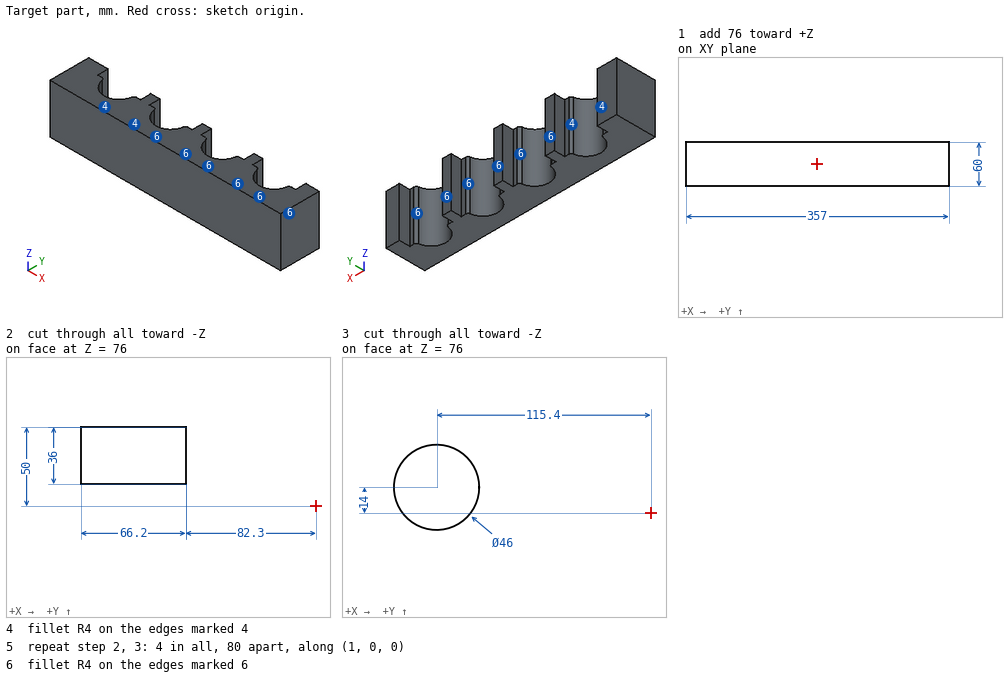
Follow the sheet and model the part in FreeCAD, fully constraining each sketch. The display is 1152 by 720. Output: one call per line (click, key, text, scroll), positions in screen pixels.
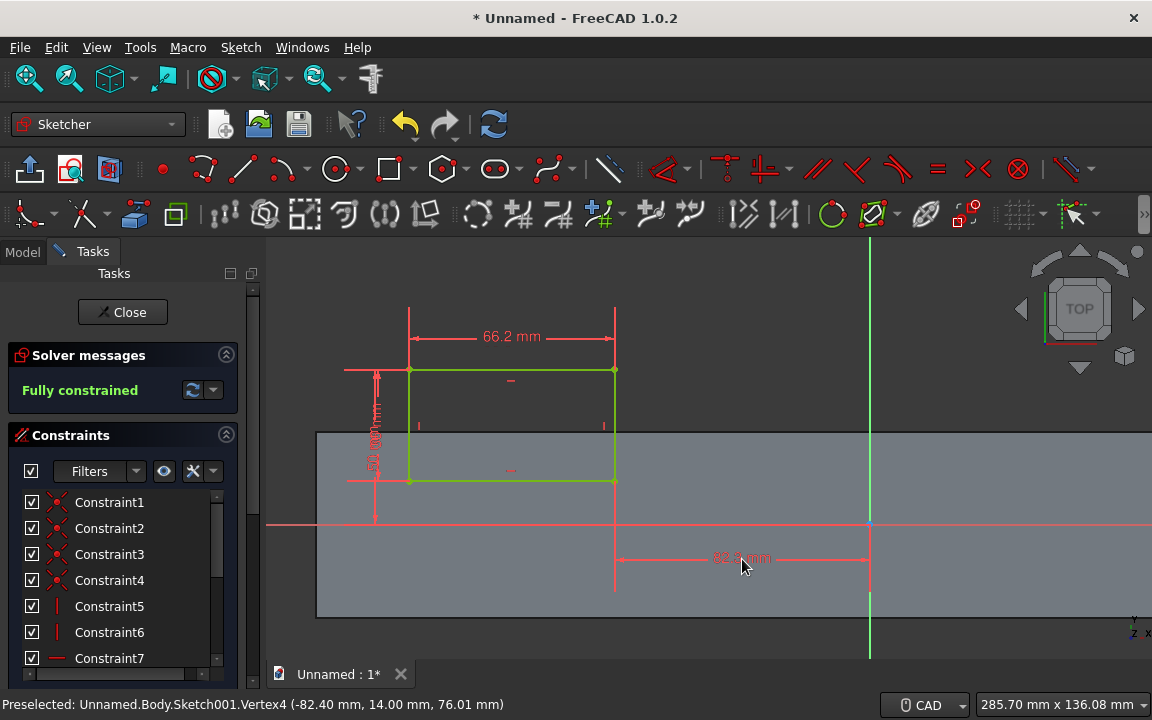
click(123, 312)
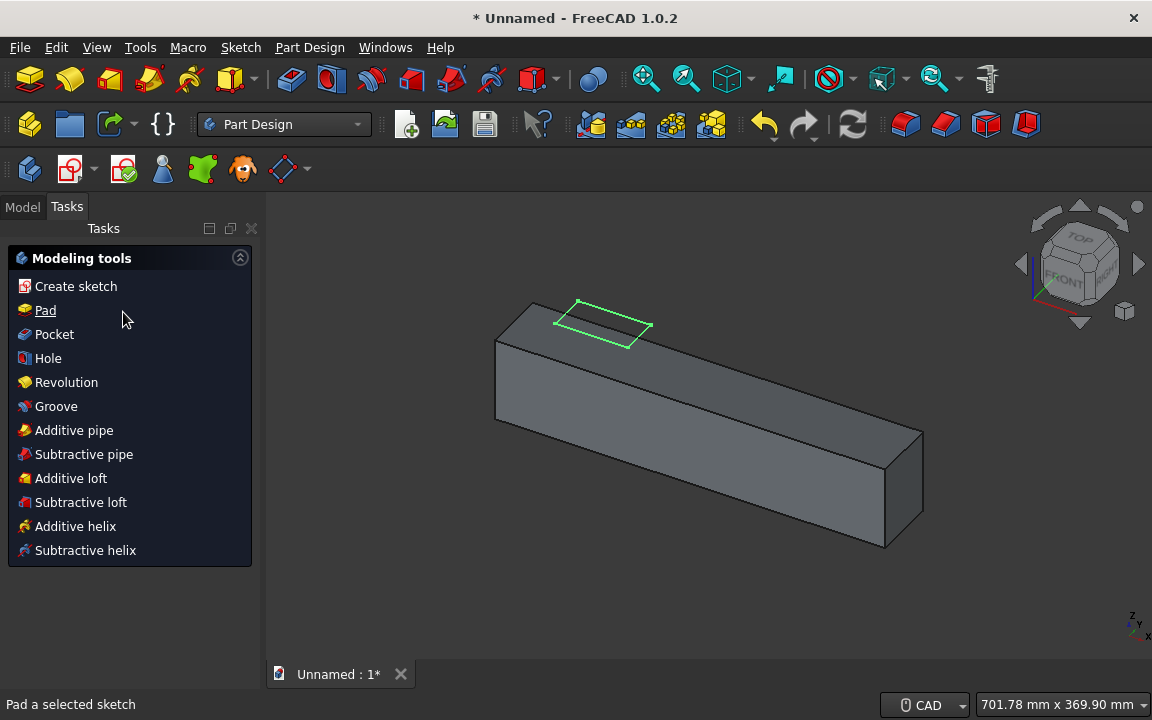
click(292, 80)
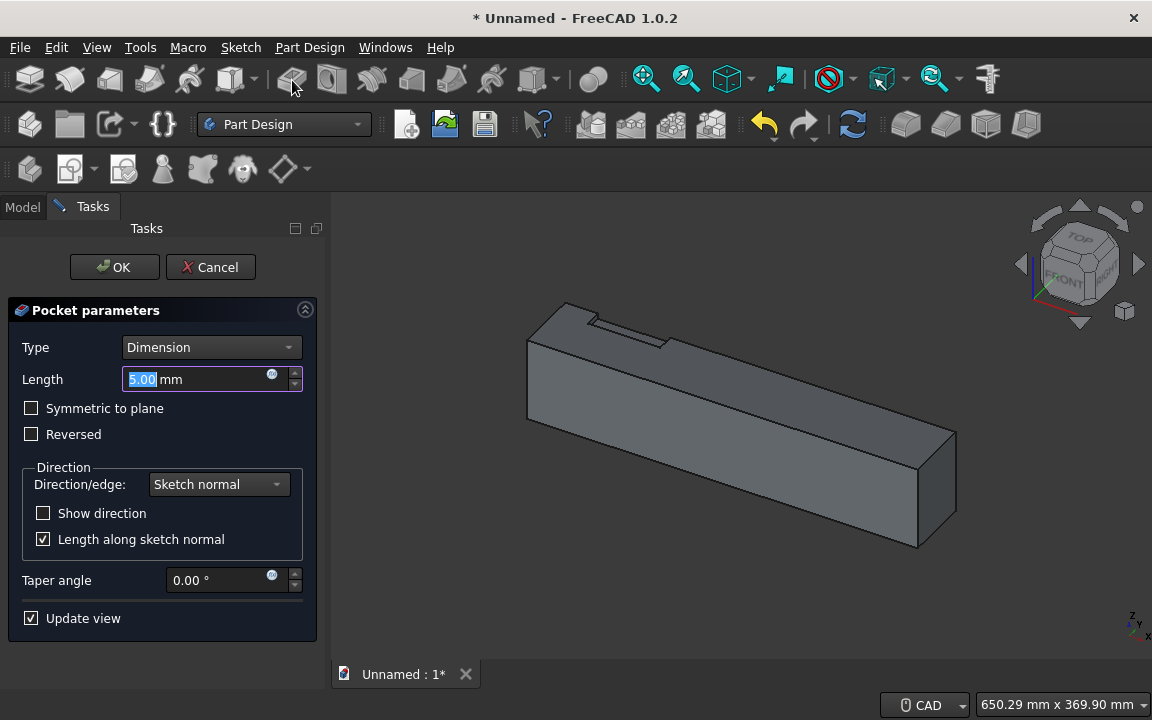
click(212, 348)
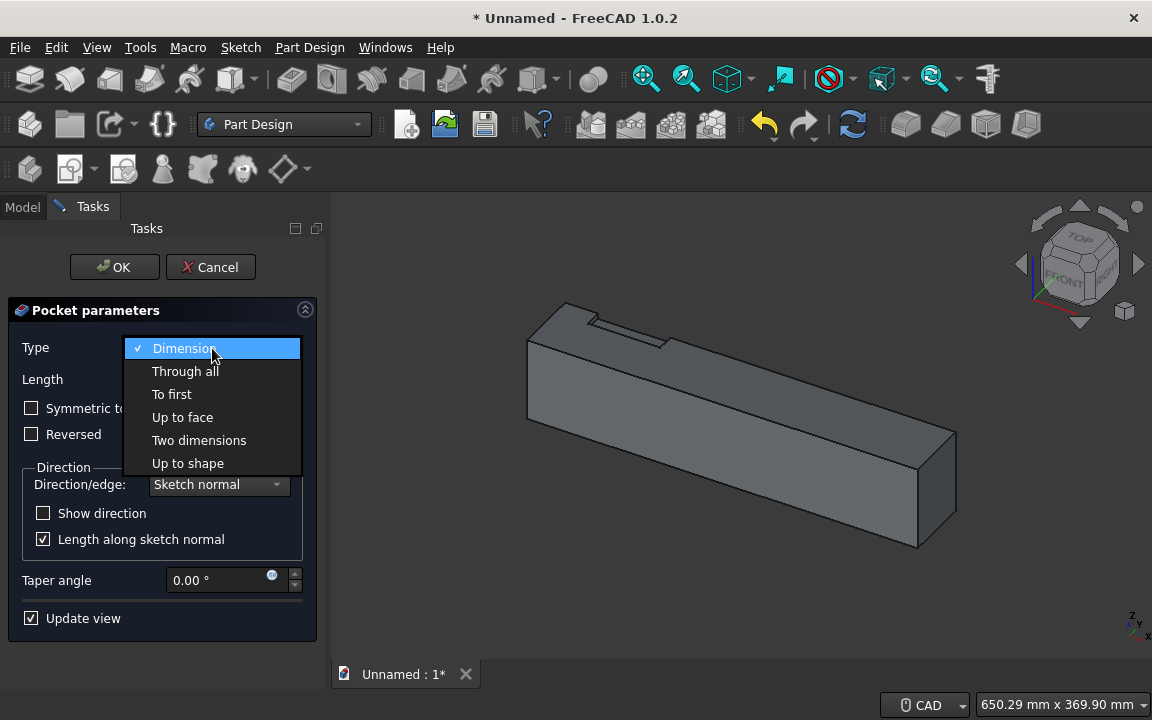
click(212, 372)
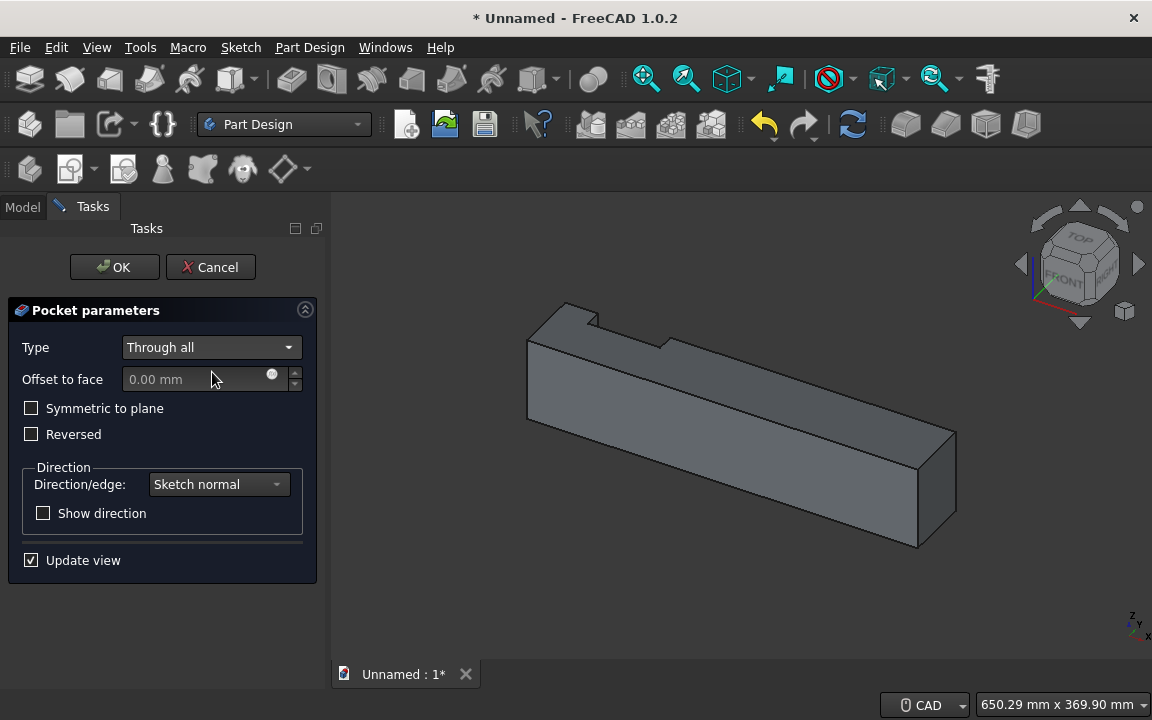
click(115, 267)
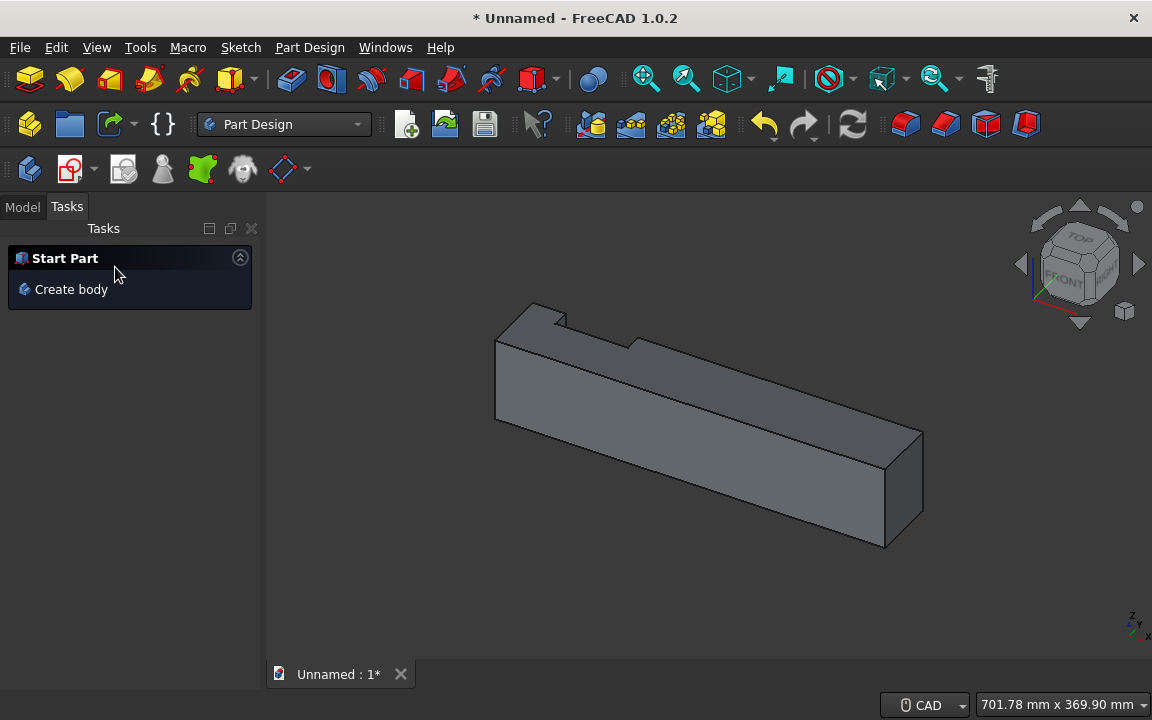
click(821, 422)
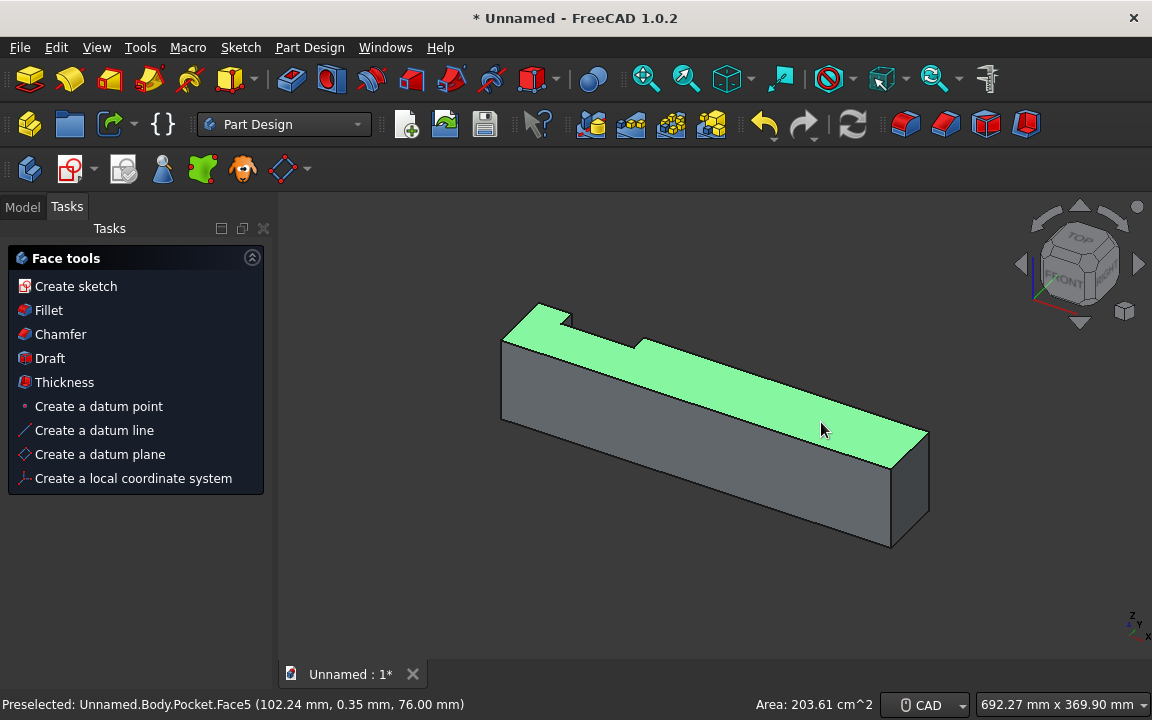
click(70, 170)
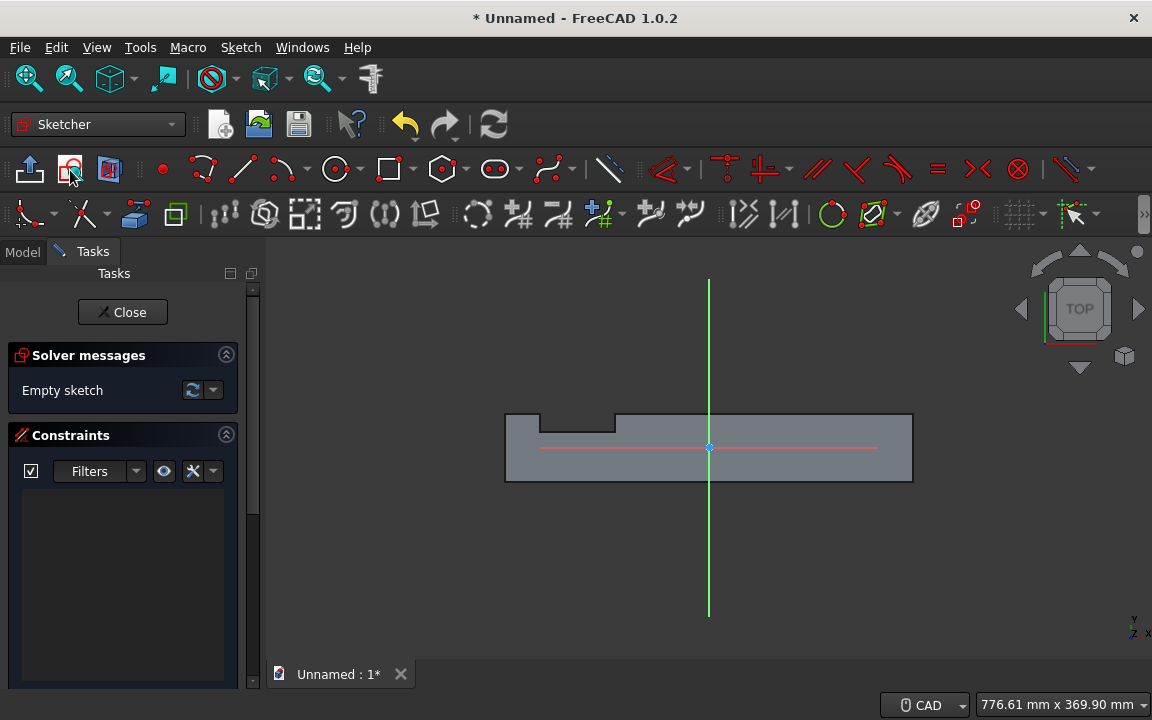
scroll(561, 428, up, 8)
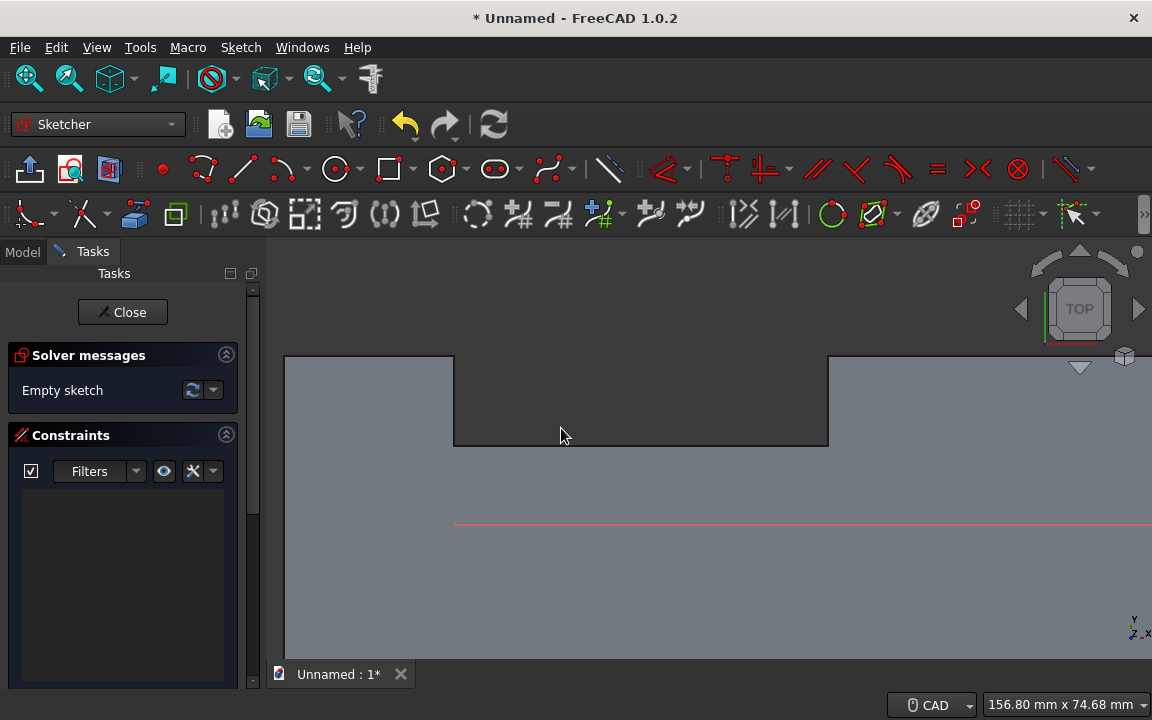
key(g)
key(c)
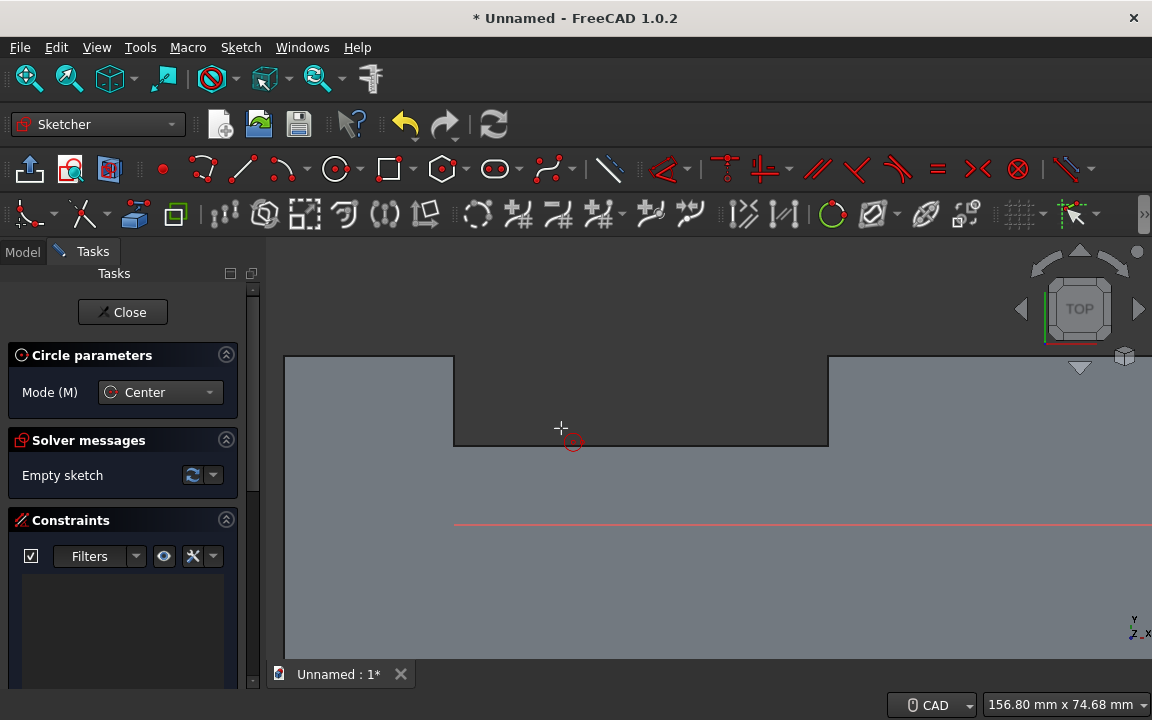
click(641, 446)
move(733, 354)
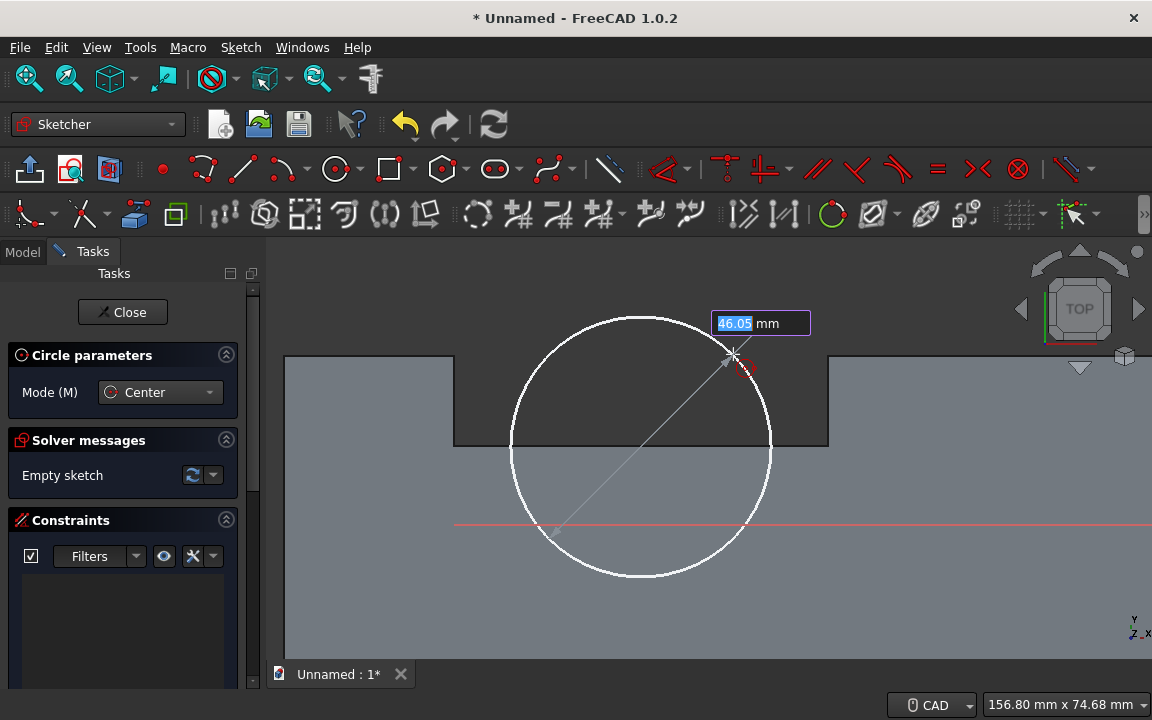
text(46)
key(Return)
key(Escape)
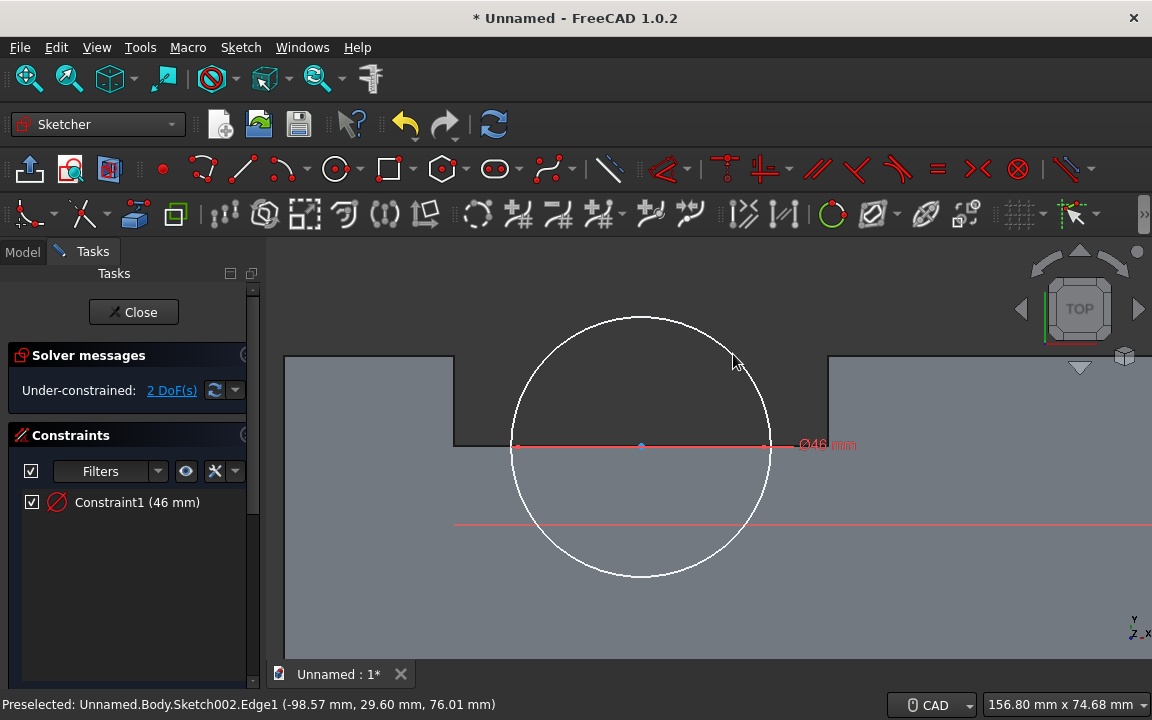
key(d)